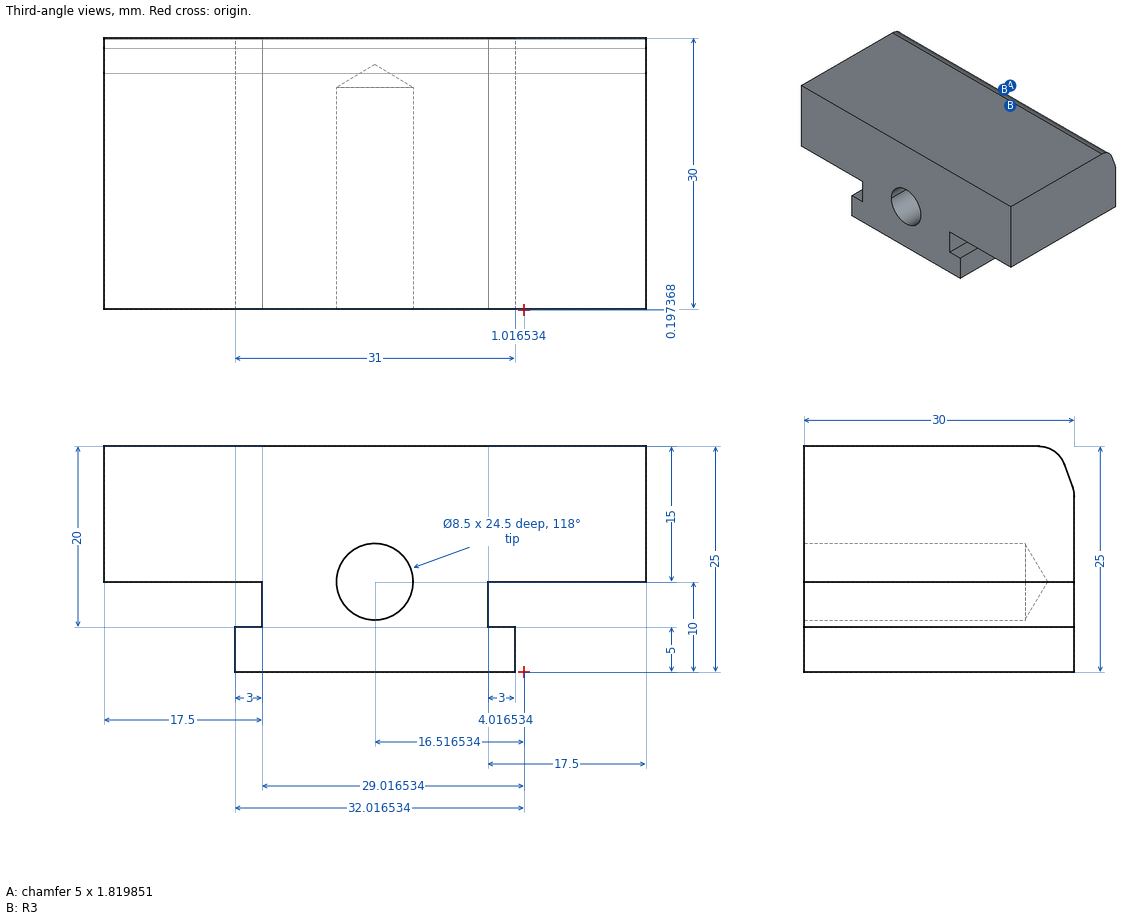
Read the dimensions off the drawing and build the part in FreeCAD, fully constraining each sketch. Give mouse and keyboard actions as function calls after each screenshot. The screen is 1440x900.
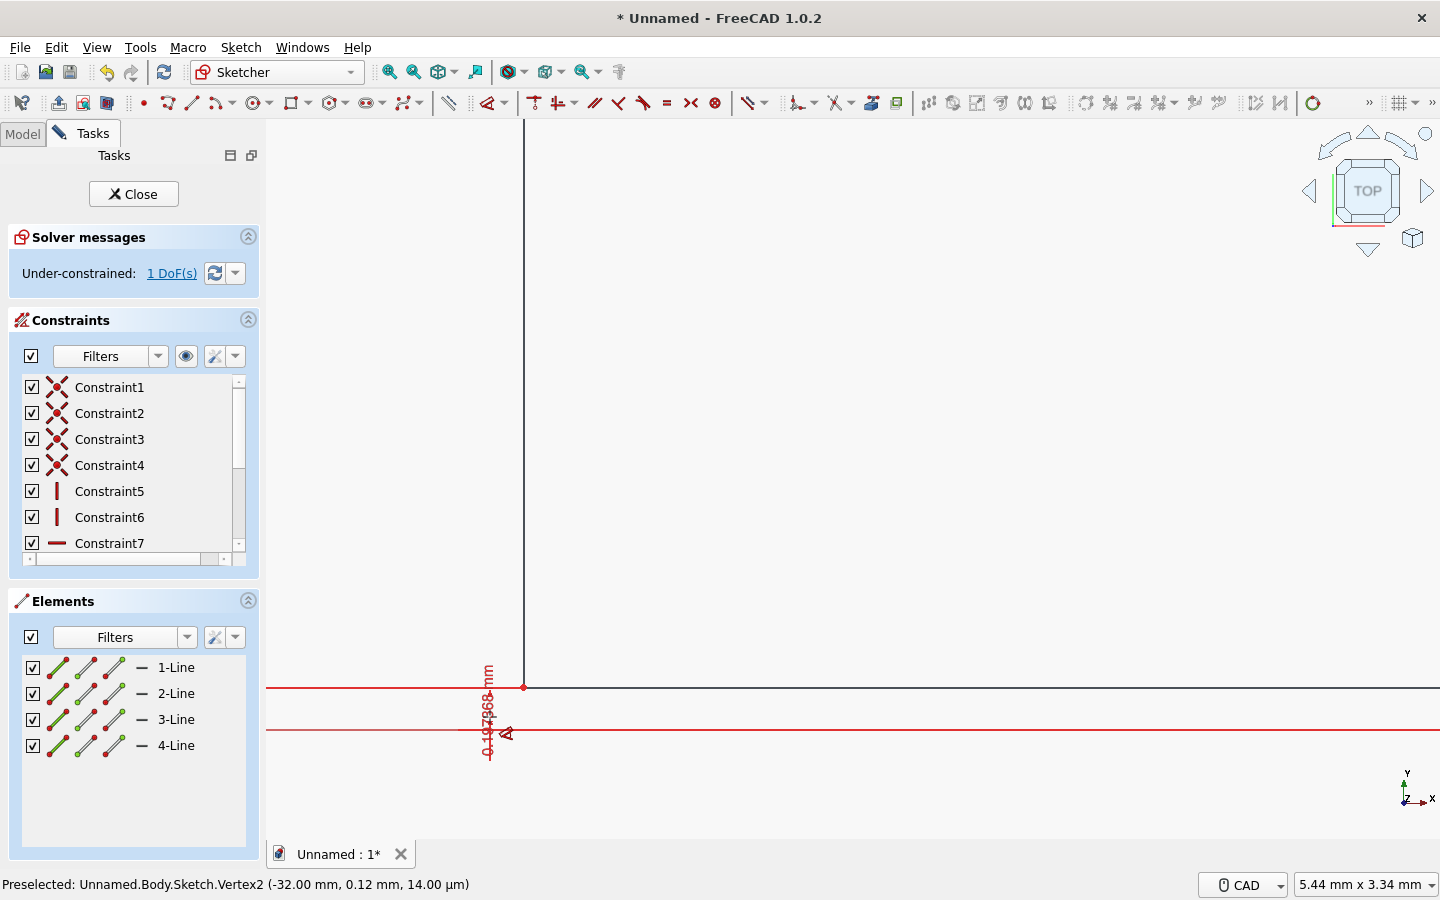
scroll(529, 720, down, 13)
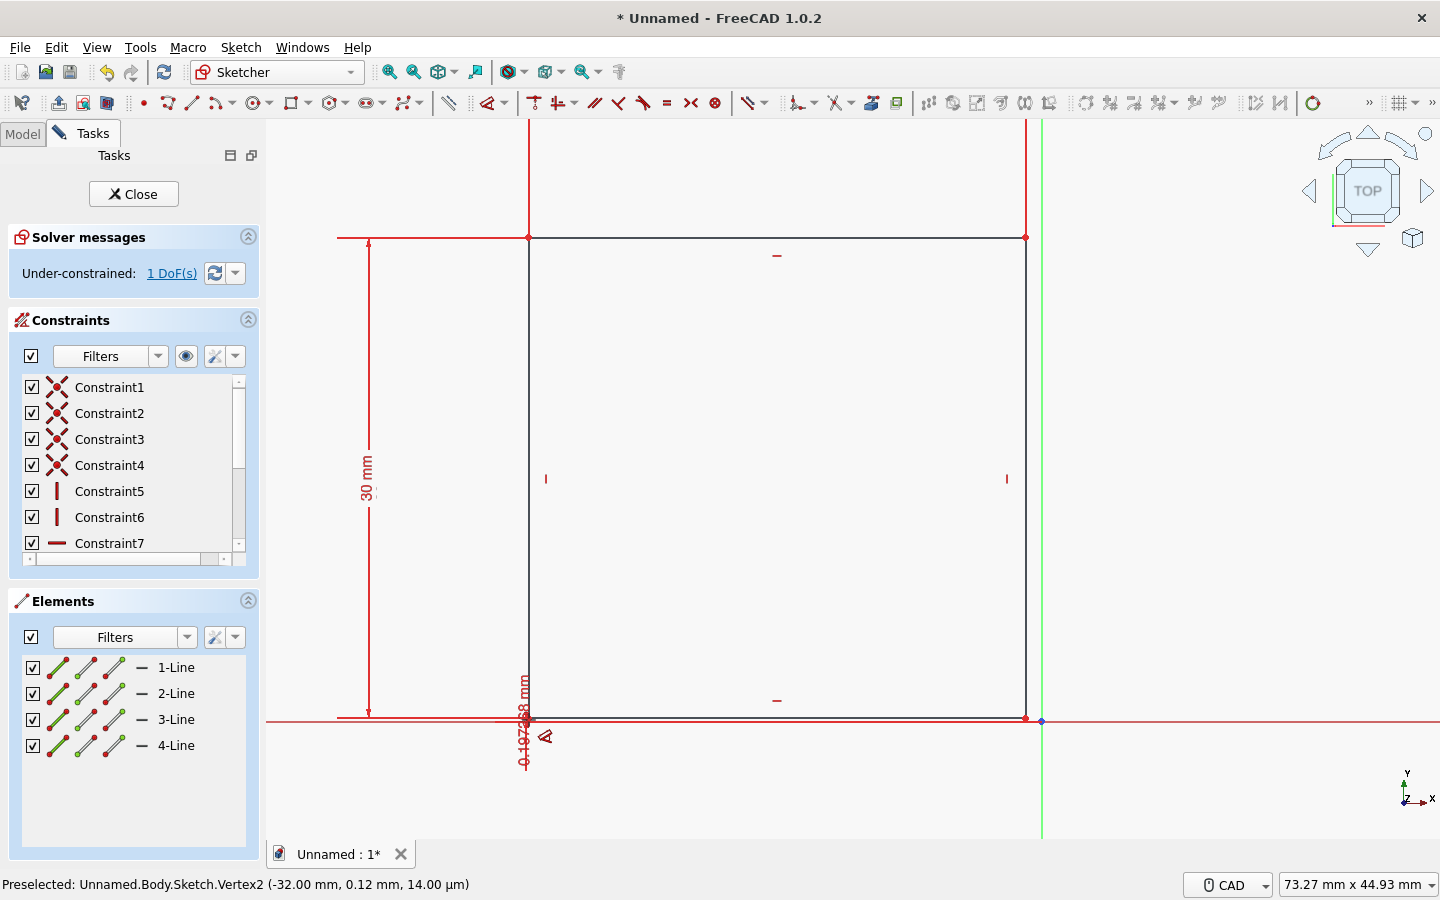
scroll(1026, 718, up, 5)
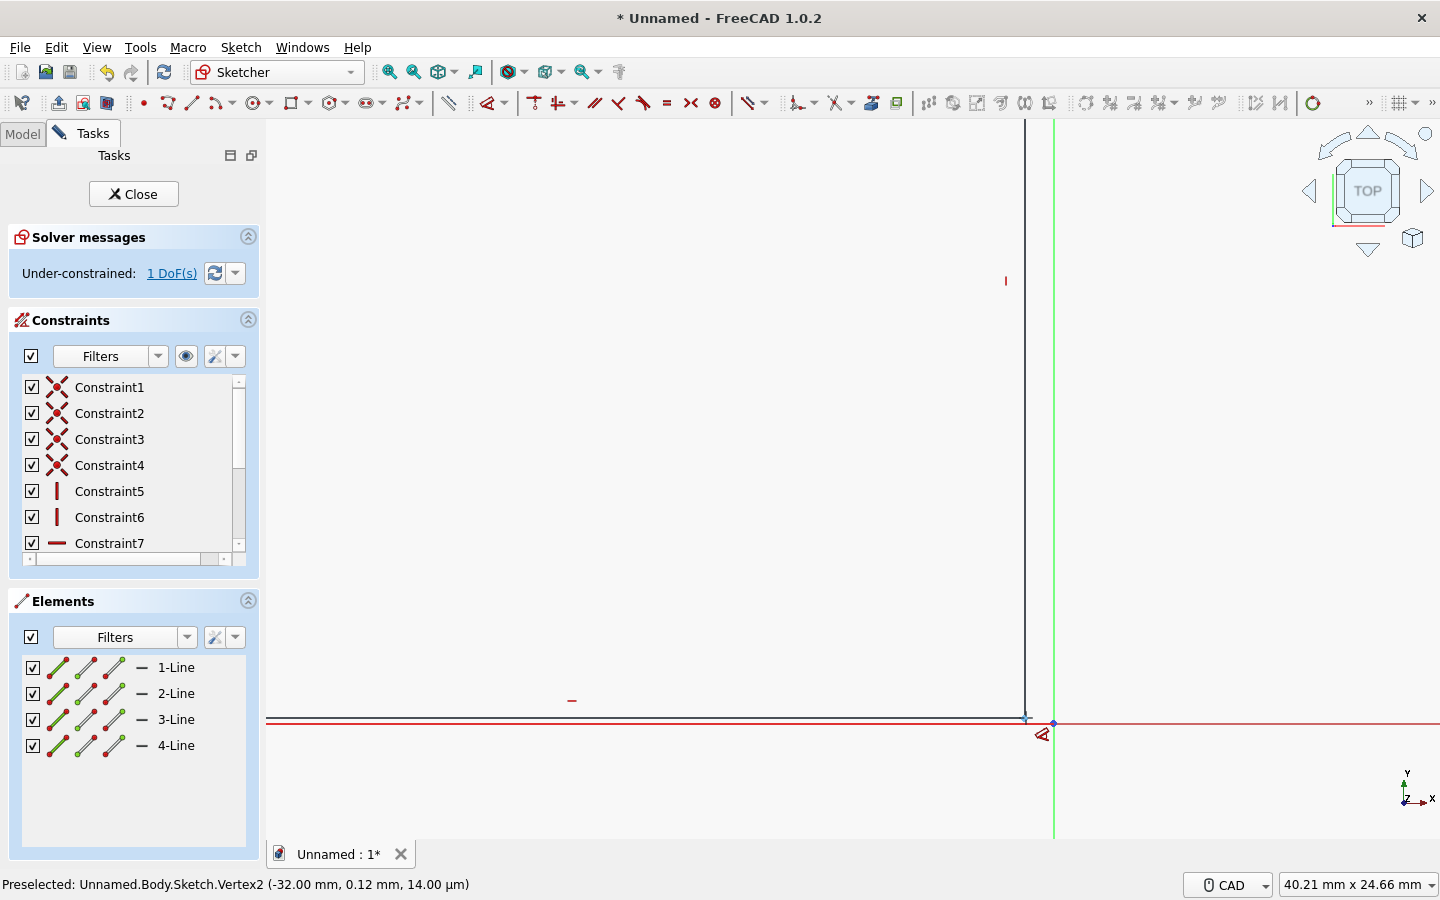
click(1024, 718)
click(1046, 760)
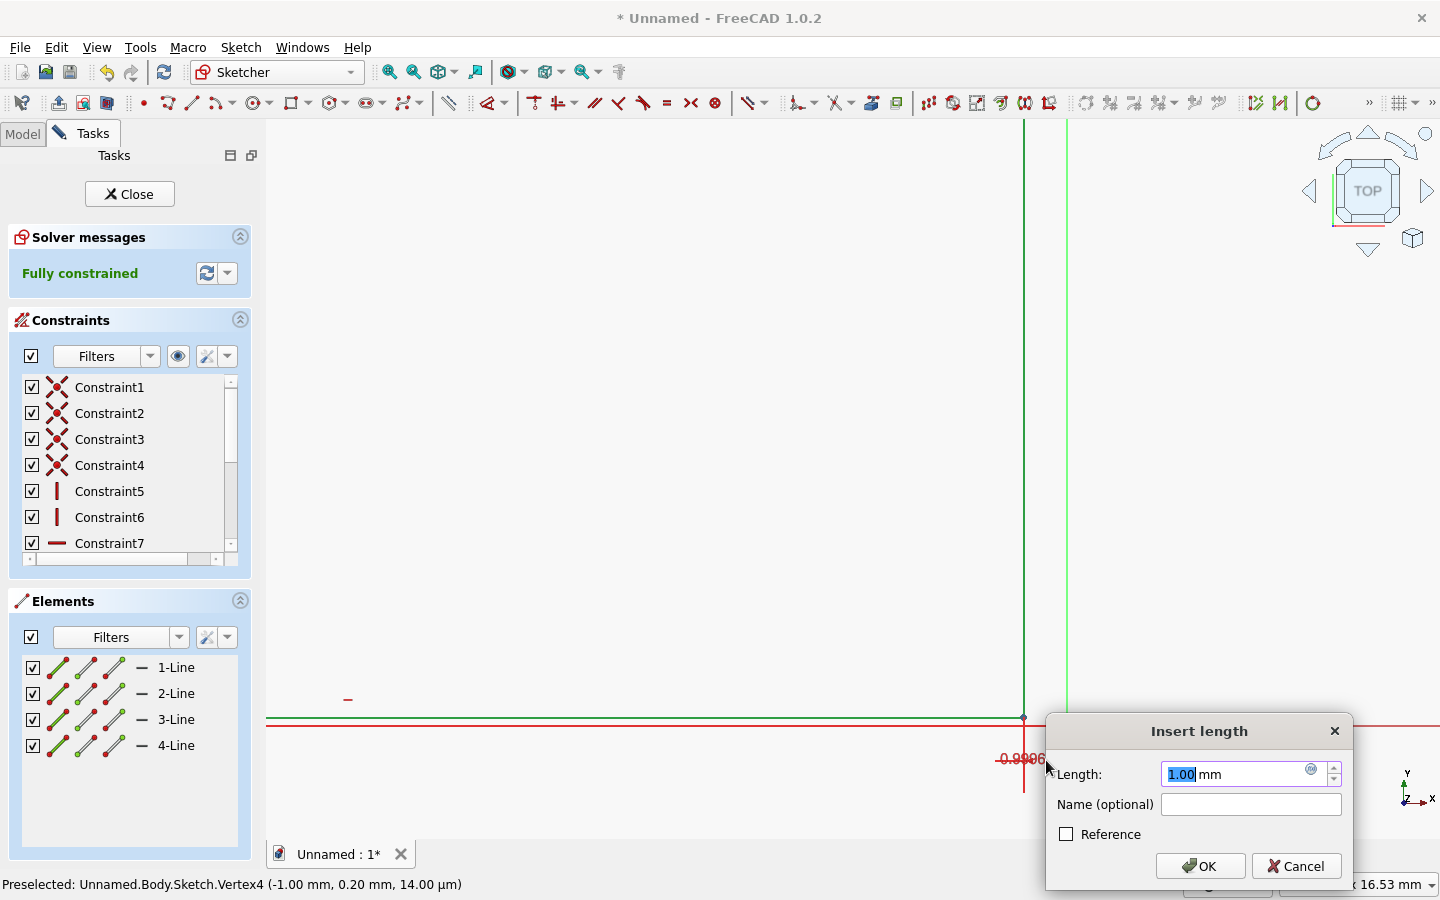
text(1.016534)
key(Return)
key(Escape)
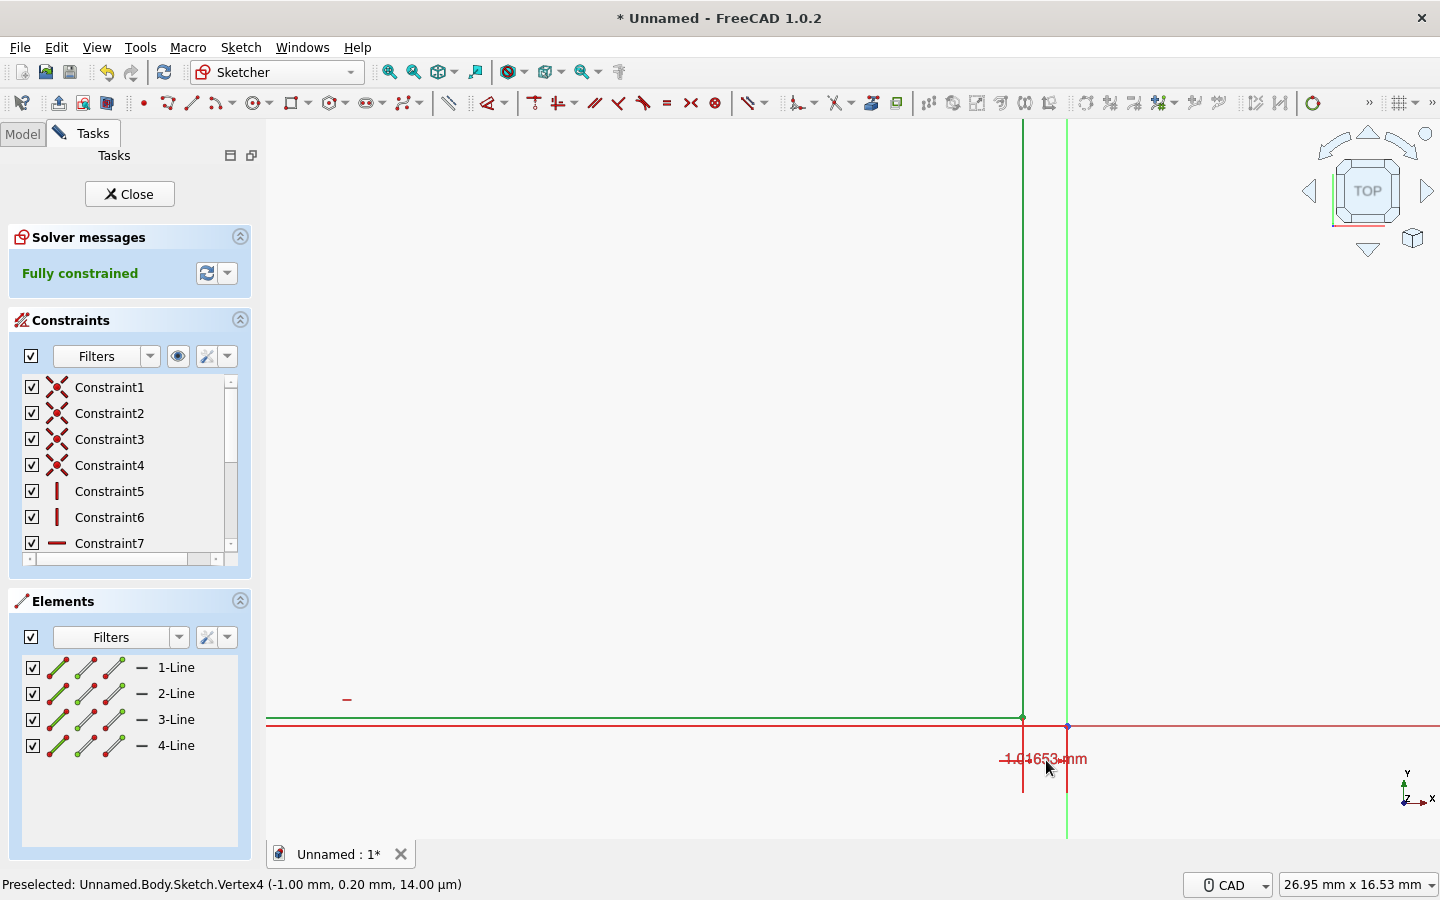
click(130, 194)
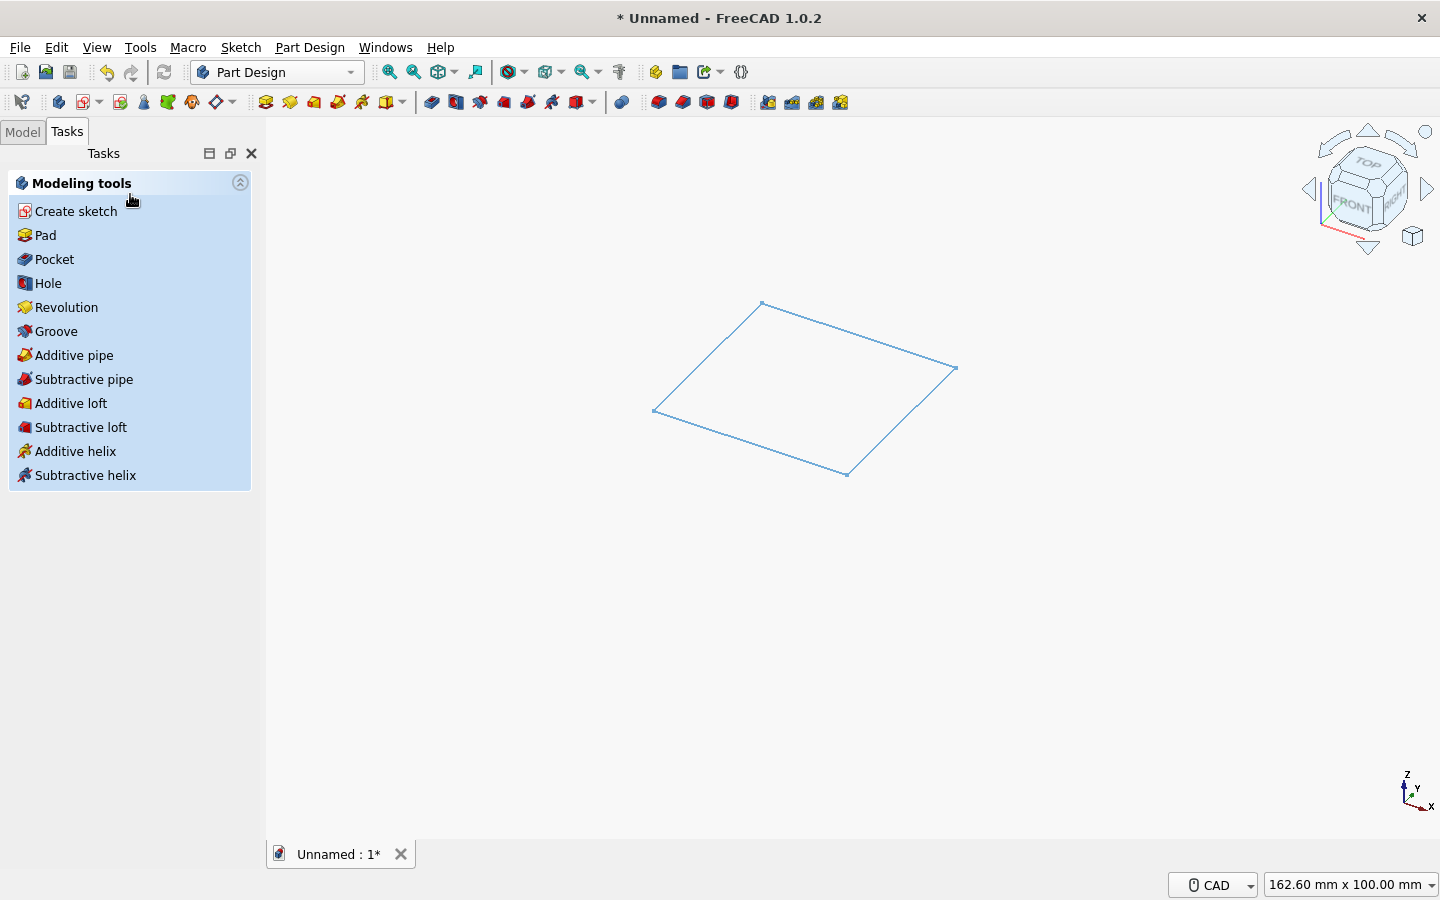
click(266, 102)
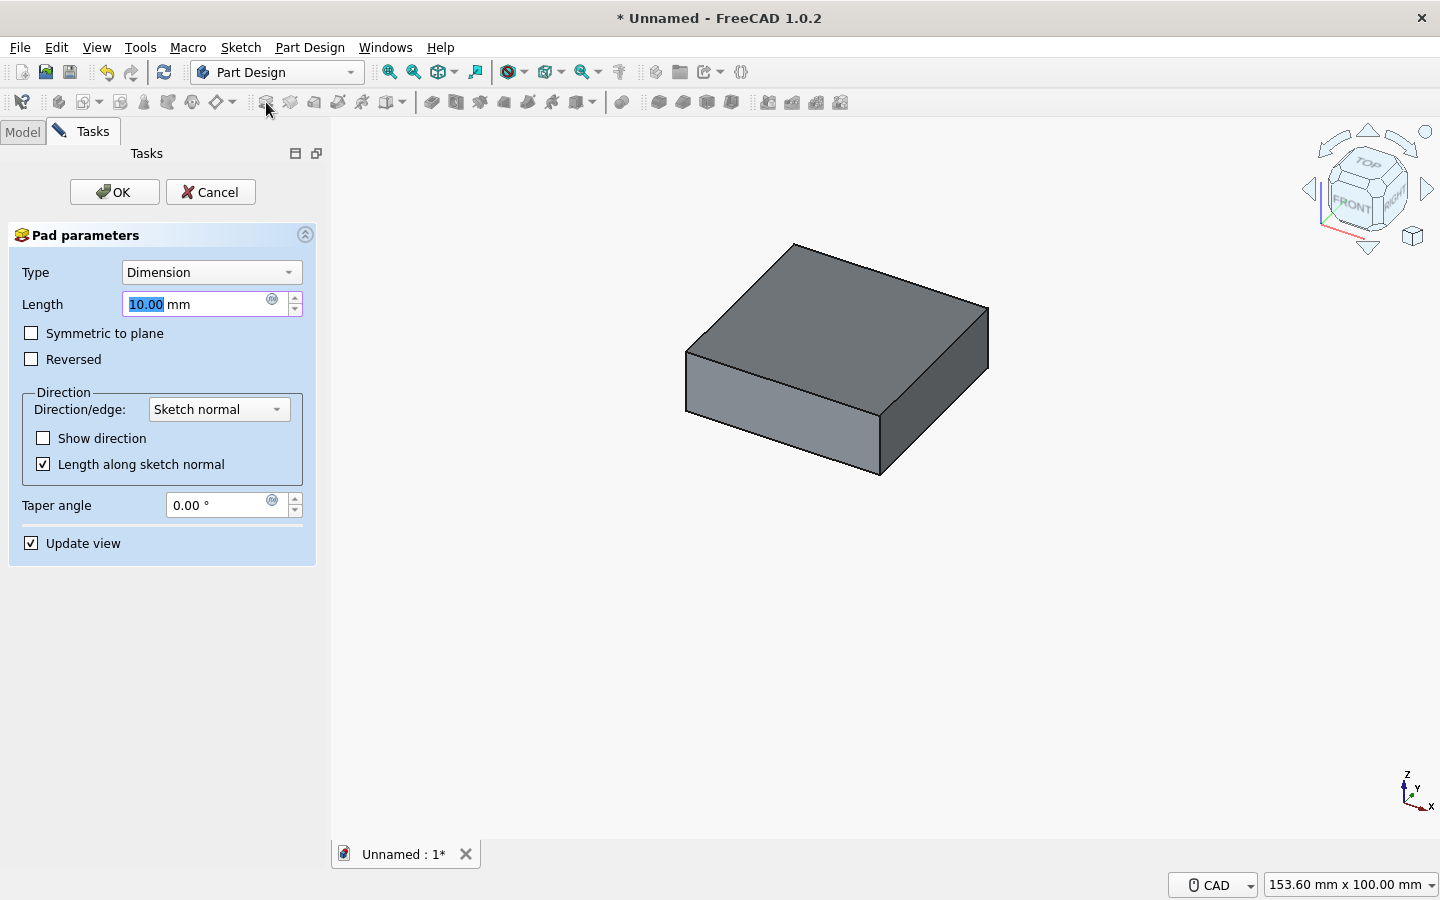
text(25)
key(Tab)